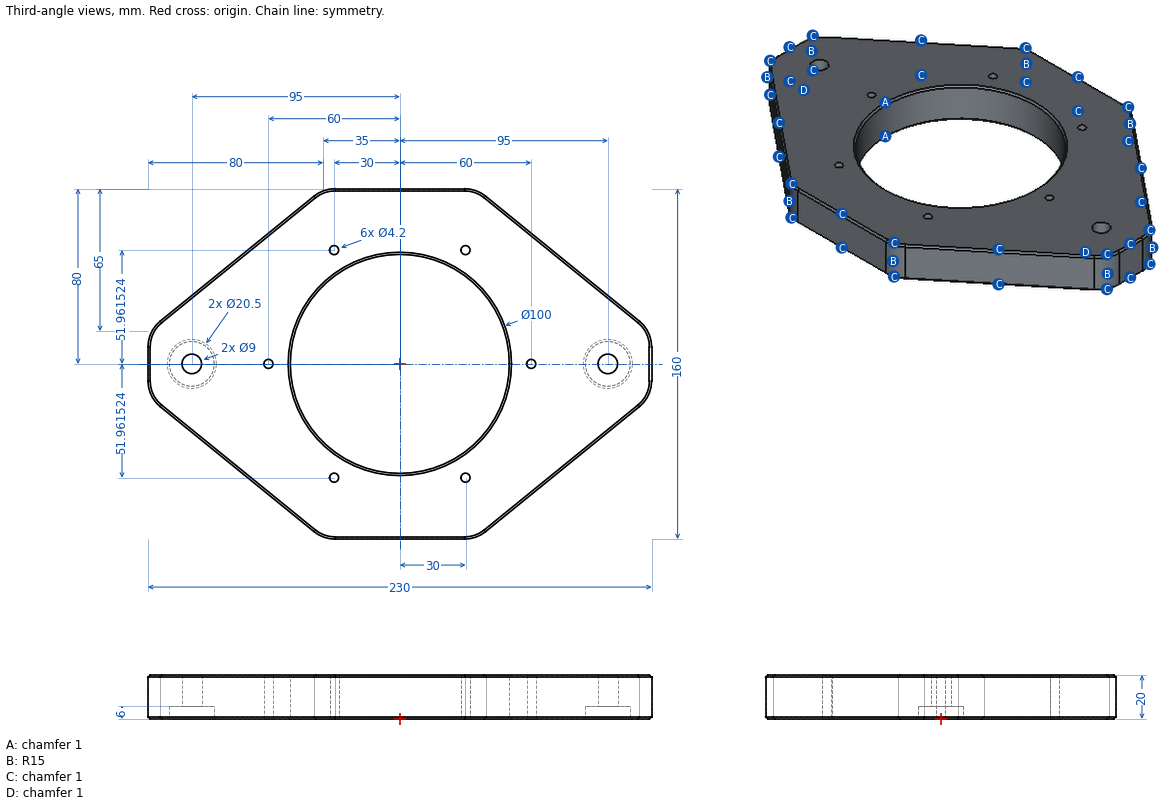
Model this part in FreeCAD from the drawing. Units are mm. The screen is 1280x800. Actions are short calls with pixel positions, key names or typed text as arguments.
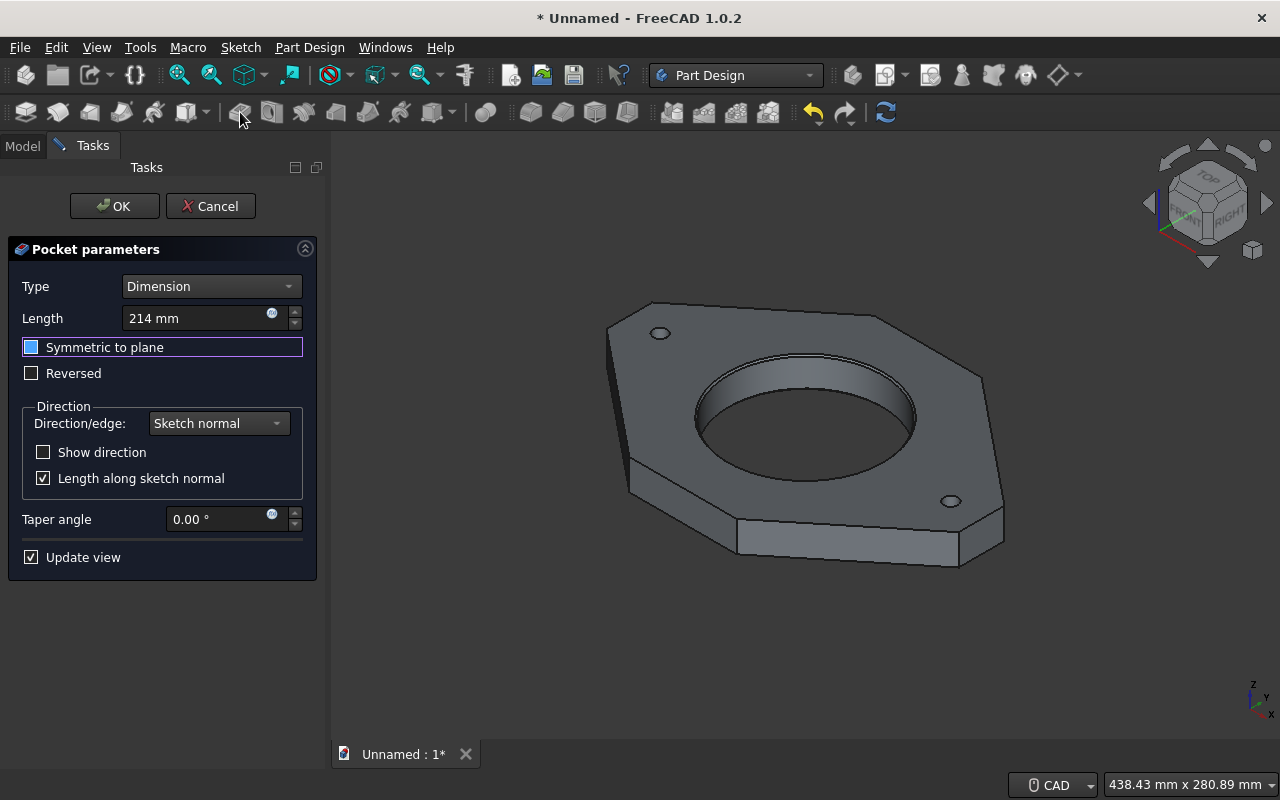
click(115, 206)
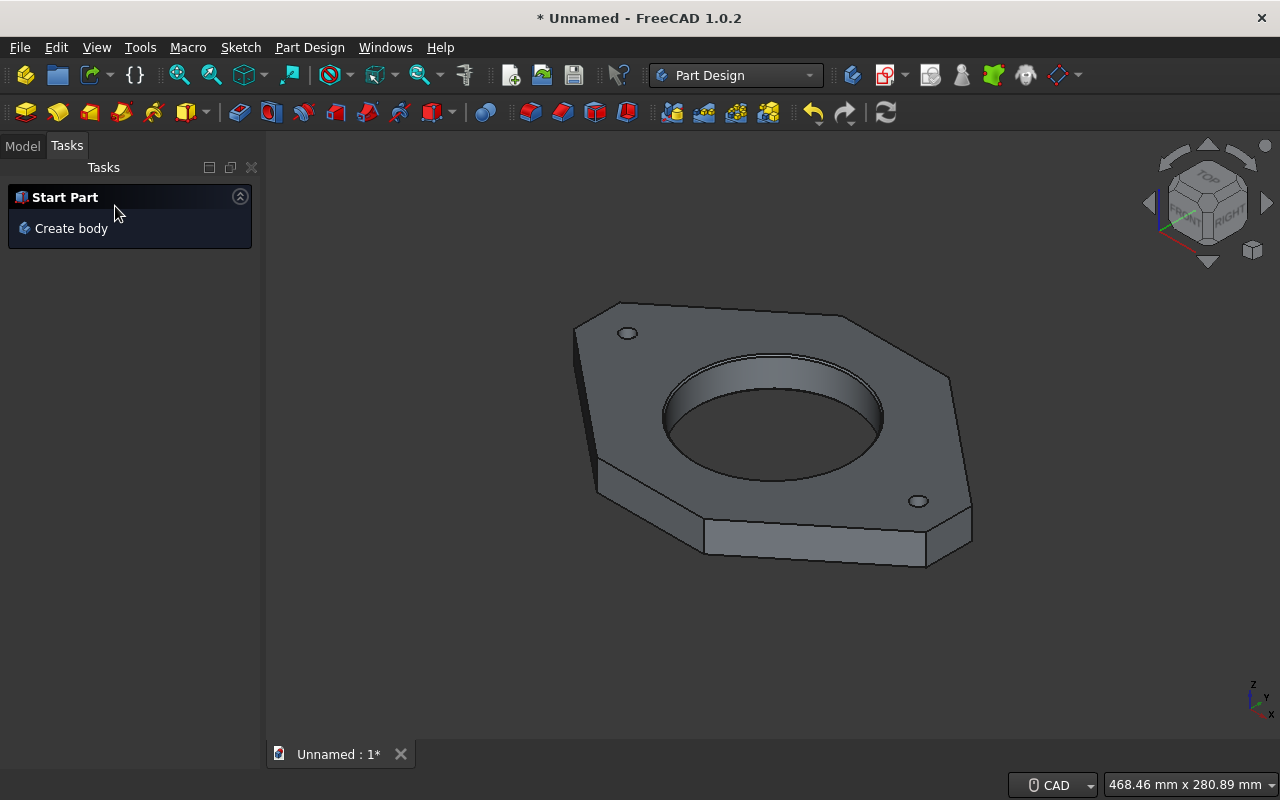
click(926, 549)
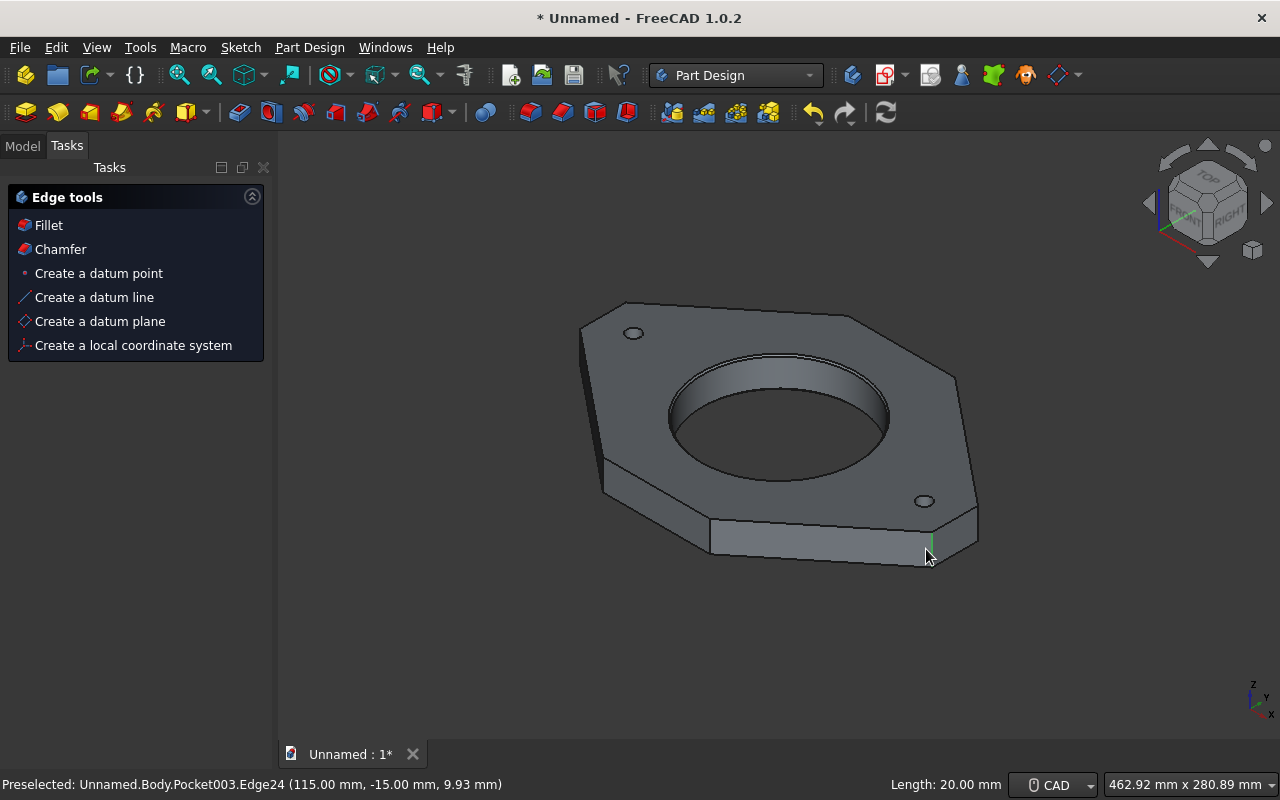
key(2)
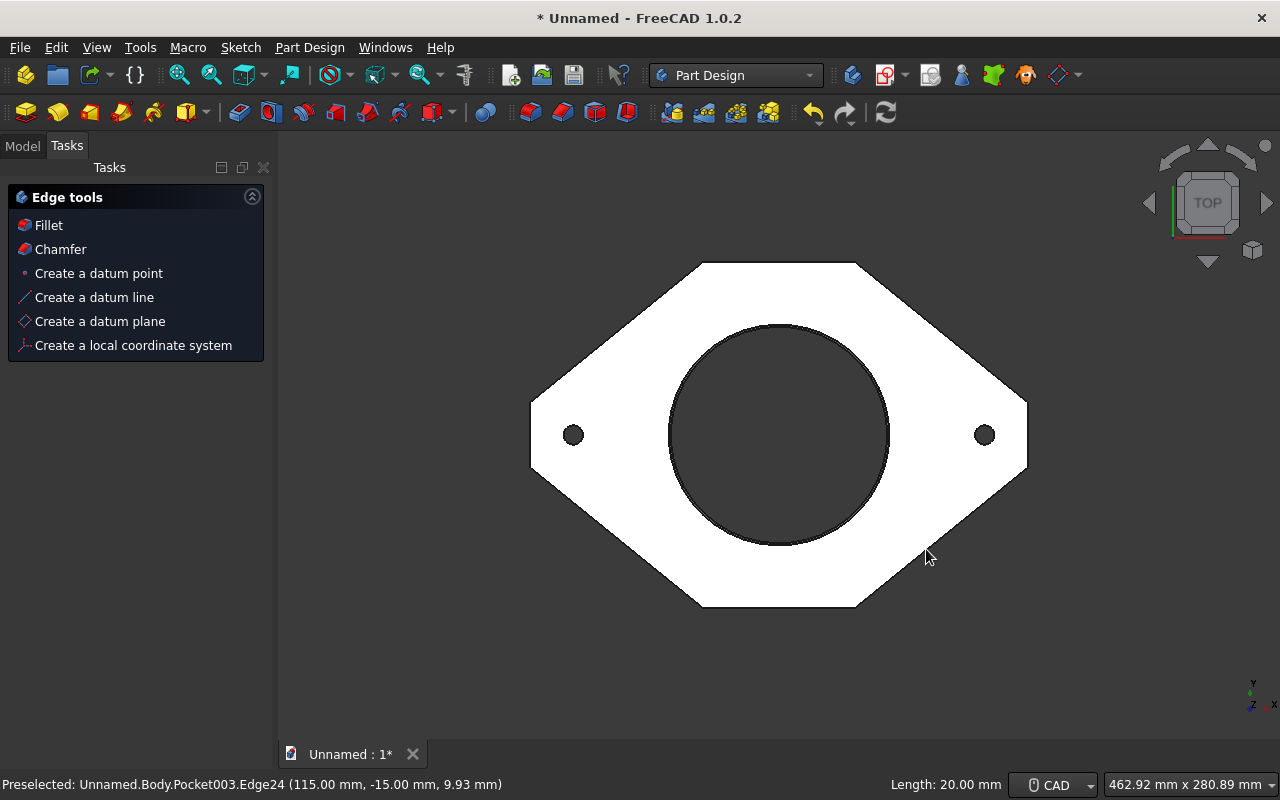
key(0)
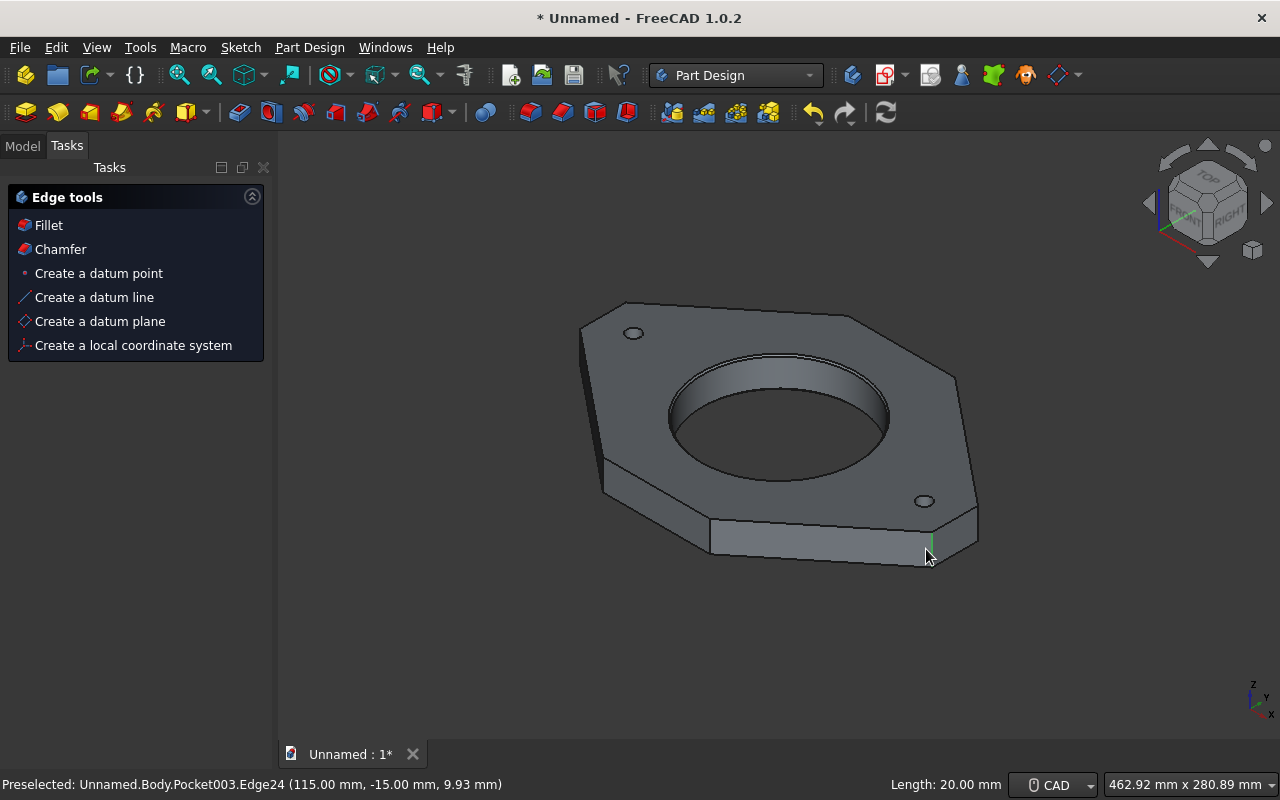
key(1)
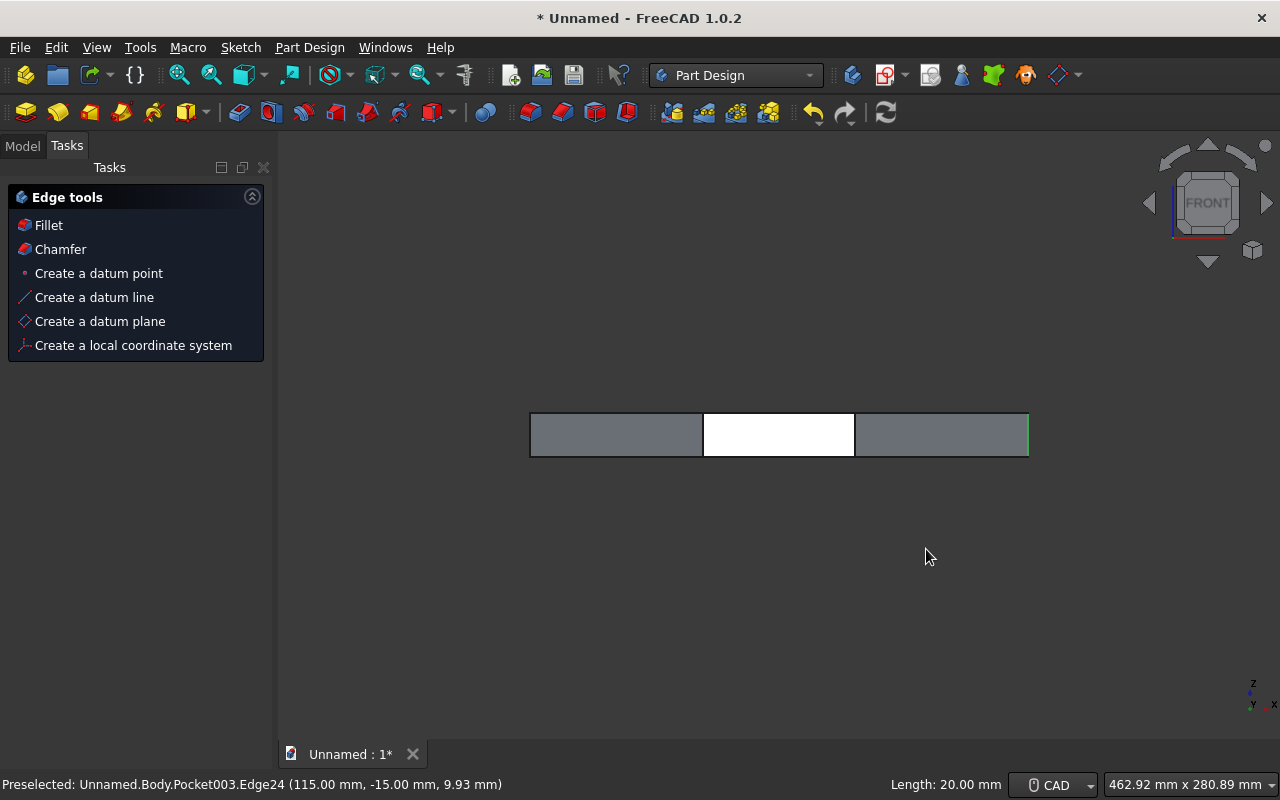
click(703, 434, ctrl)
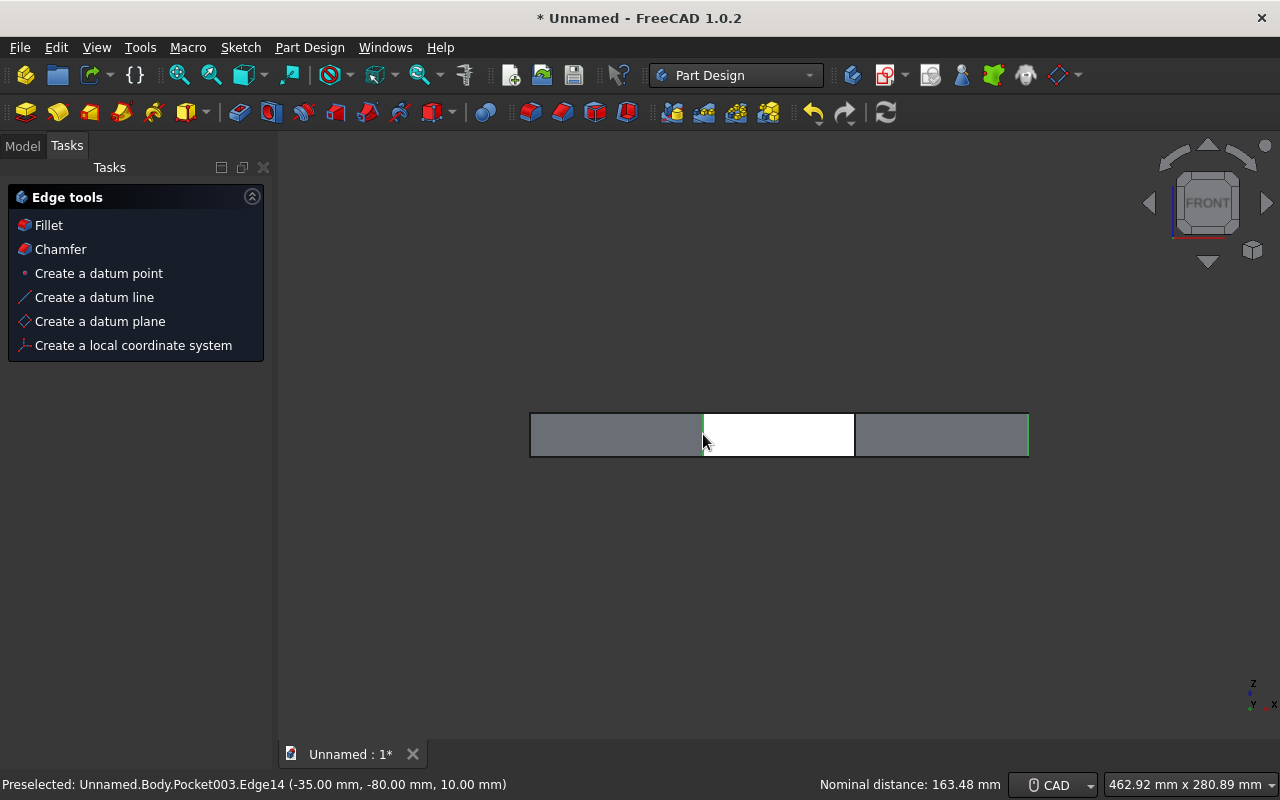
click(855, 434, ctrl)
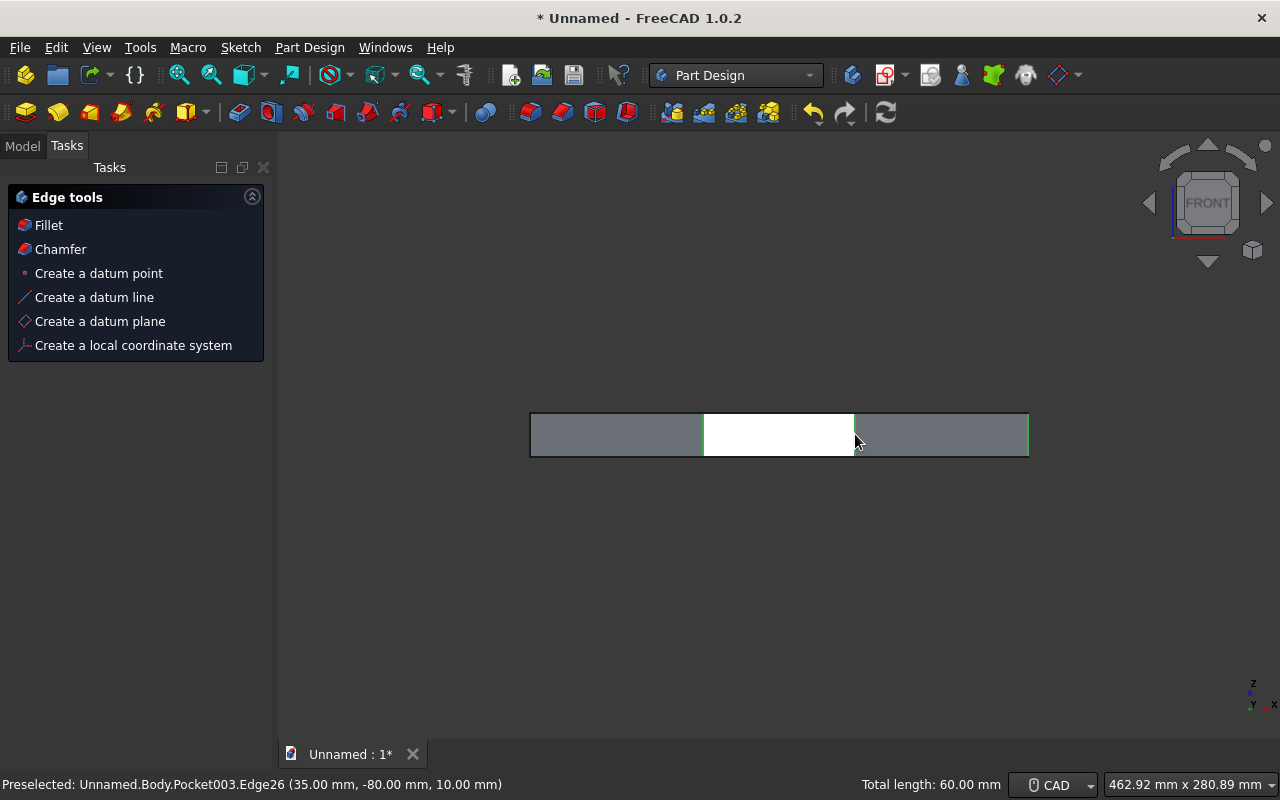
key(3)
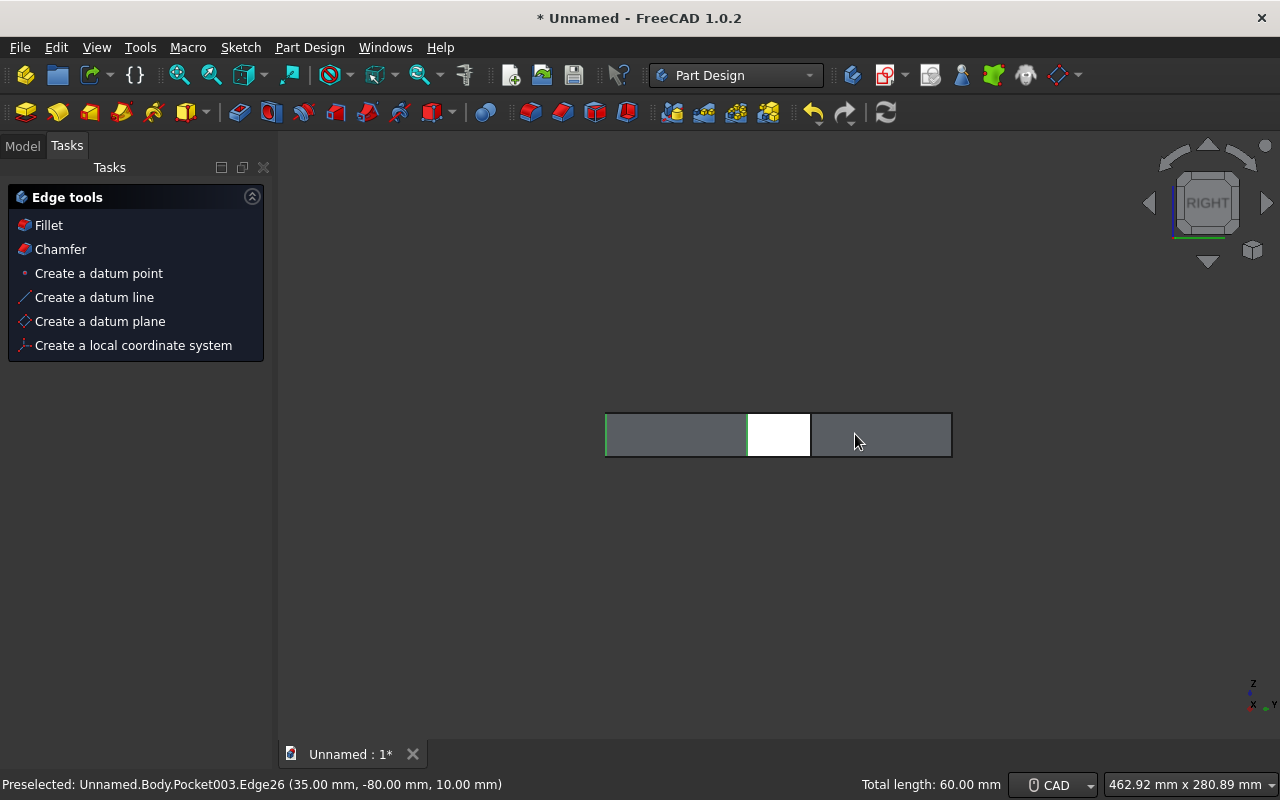
click(180, 76)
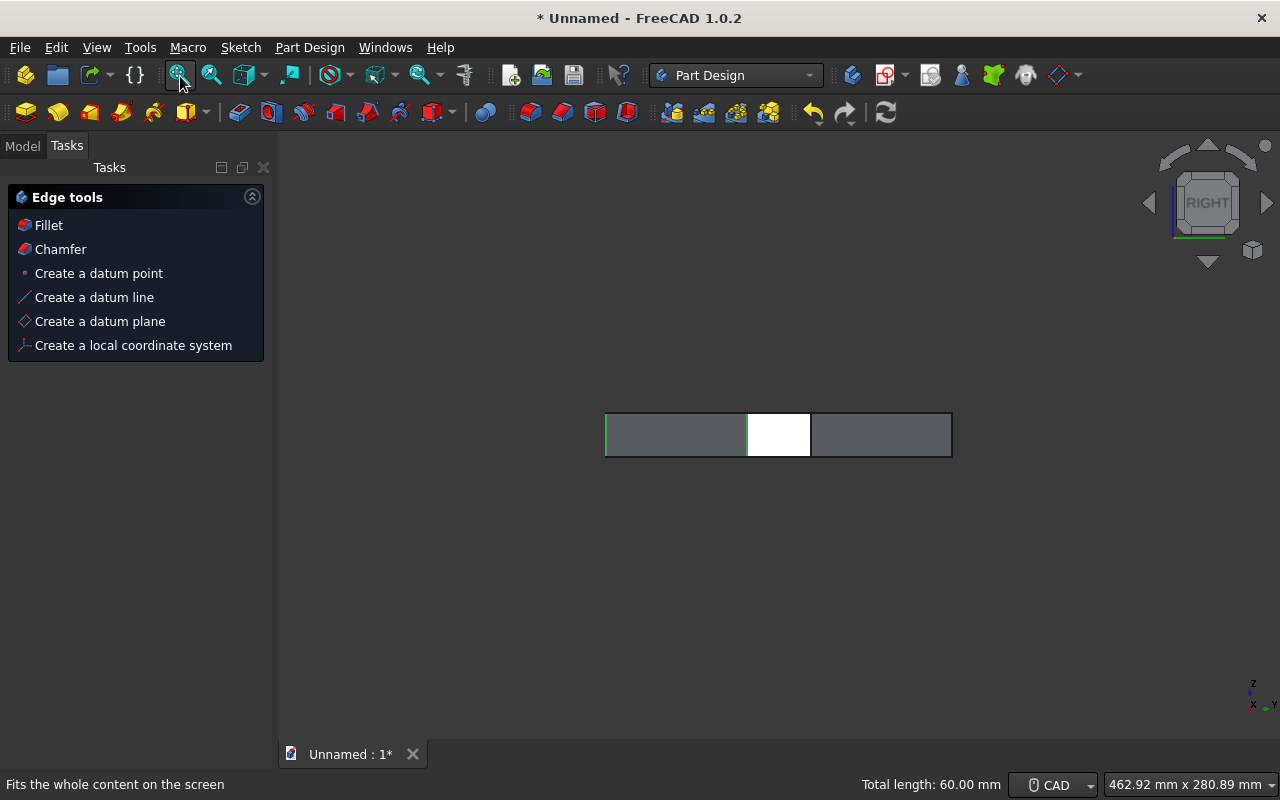
click(811, 434, ctrl)